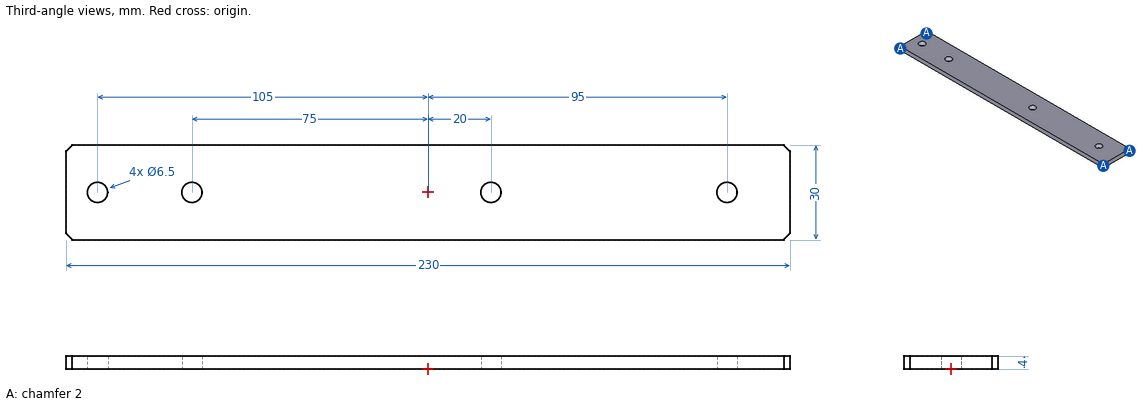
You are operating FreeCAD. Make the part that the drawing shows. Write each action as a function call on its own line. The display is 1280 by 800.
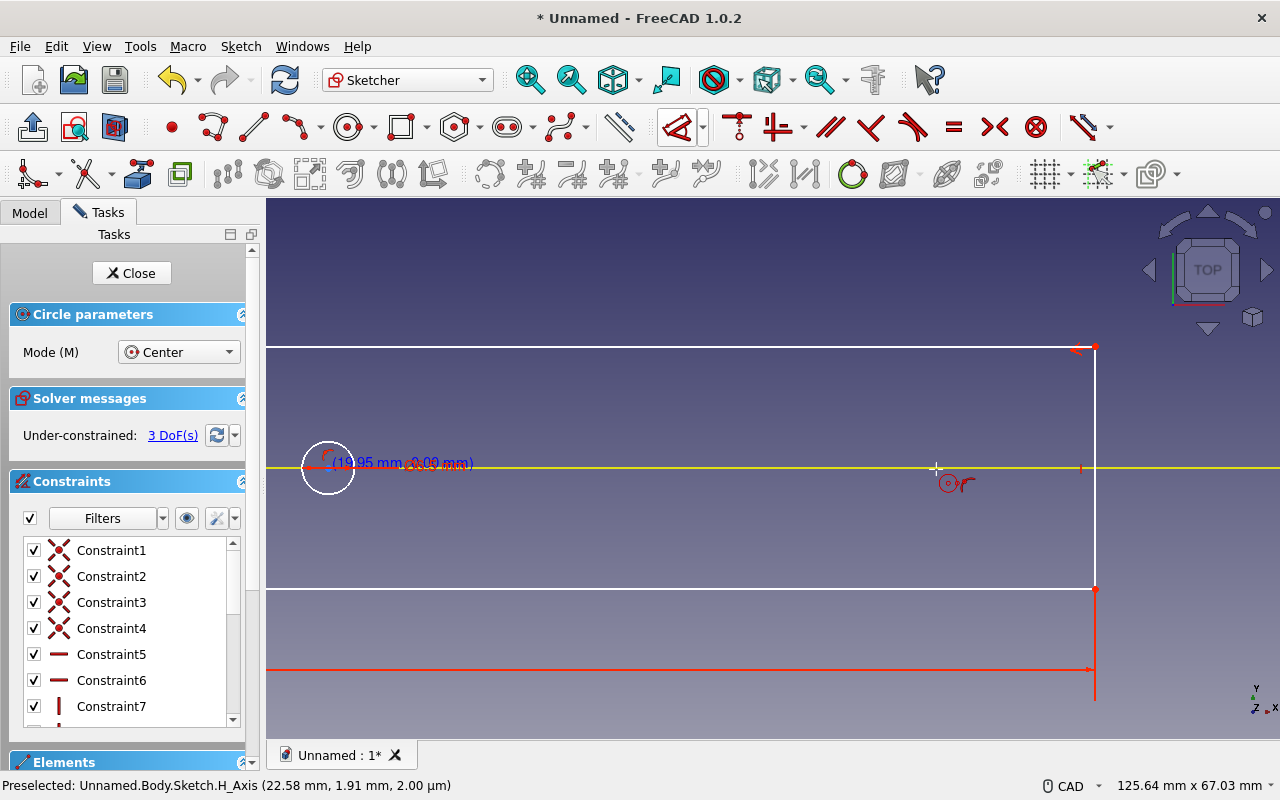
click(934, 468)
move(953, 449)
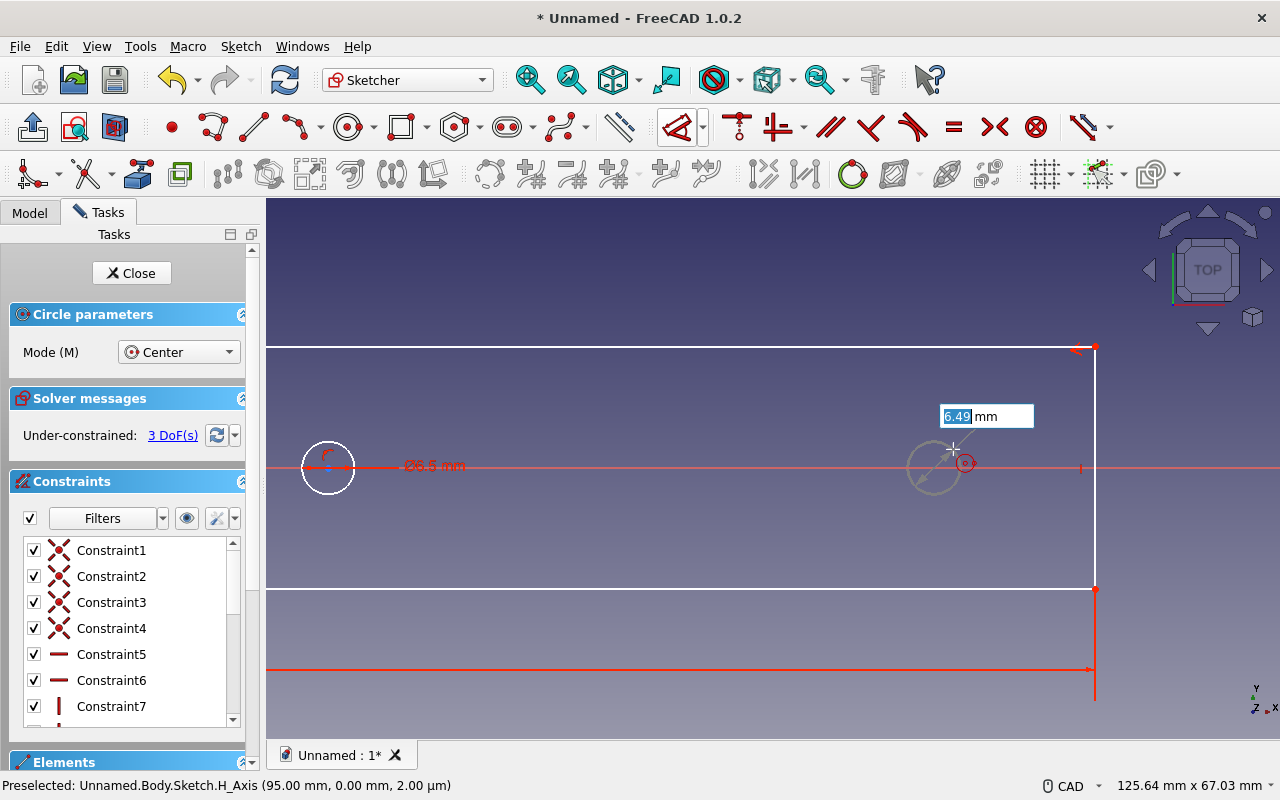
text(6.5)
key(Return)
key(Escape)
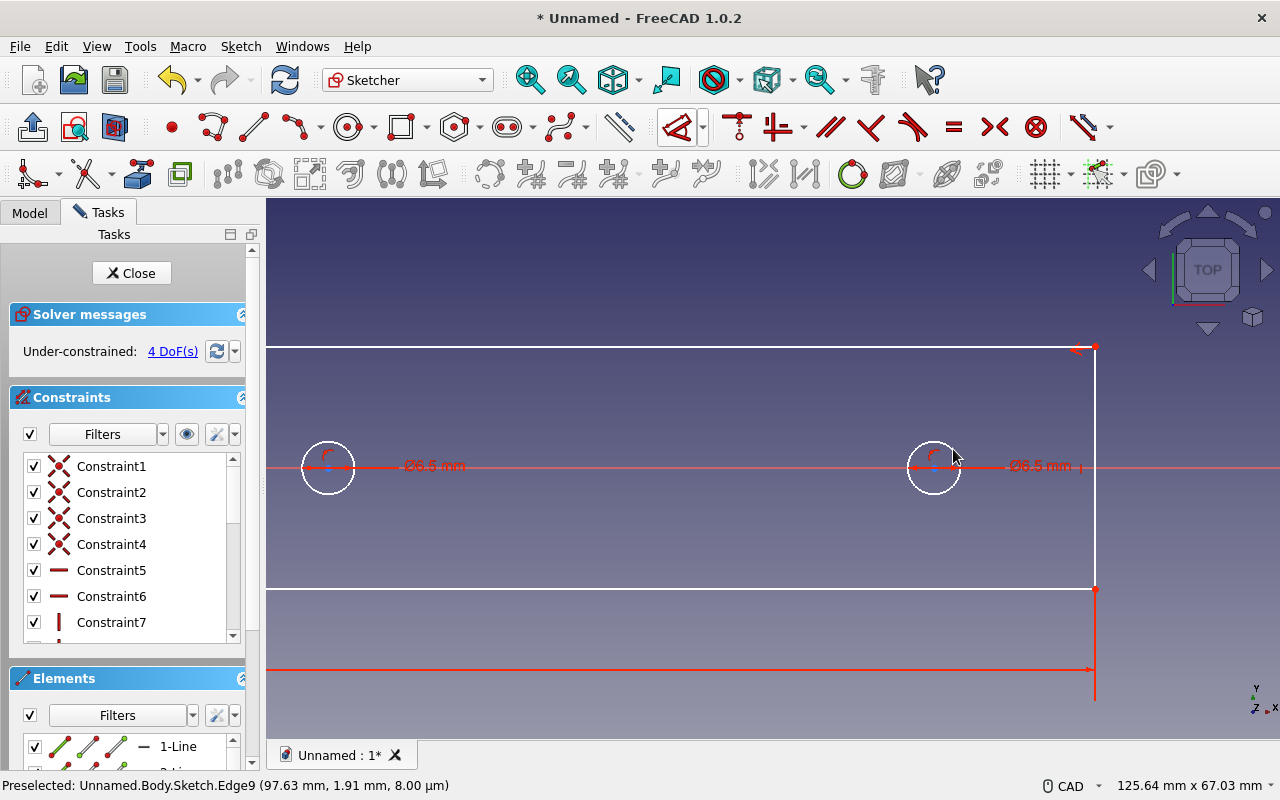
key(d)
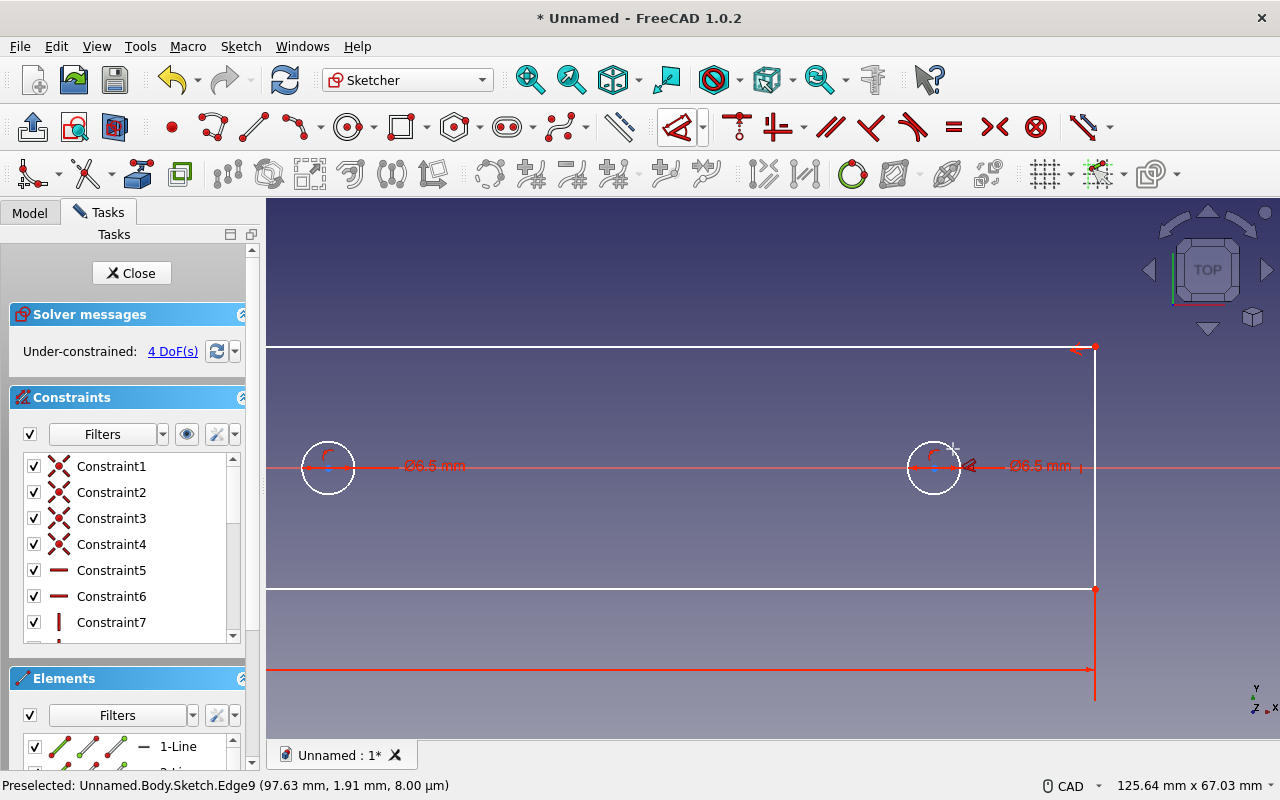
scroll(936, 469, down, 6)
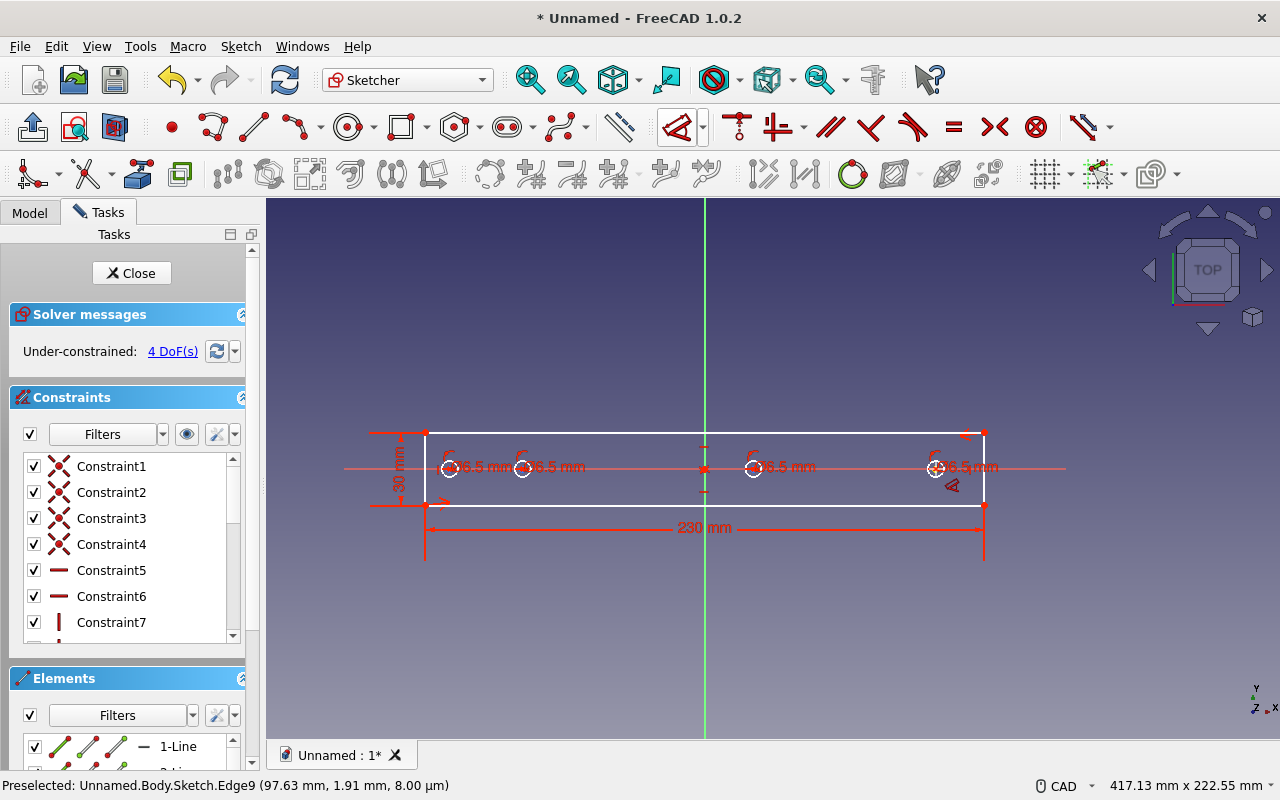
click(523, 469)
click(614, 527)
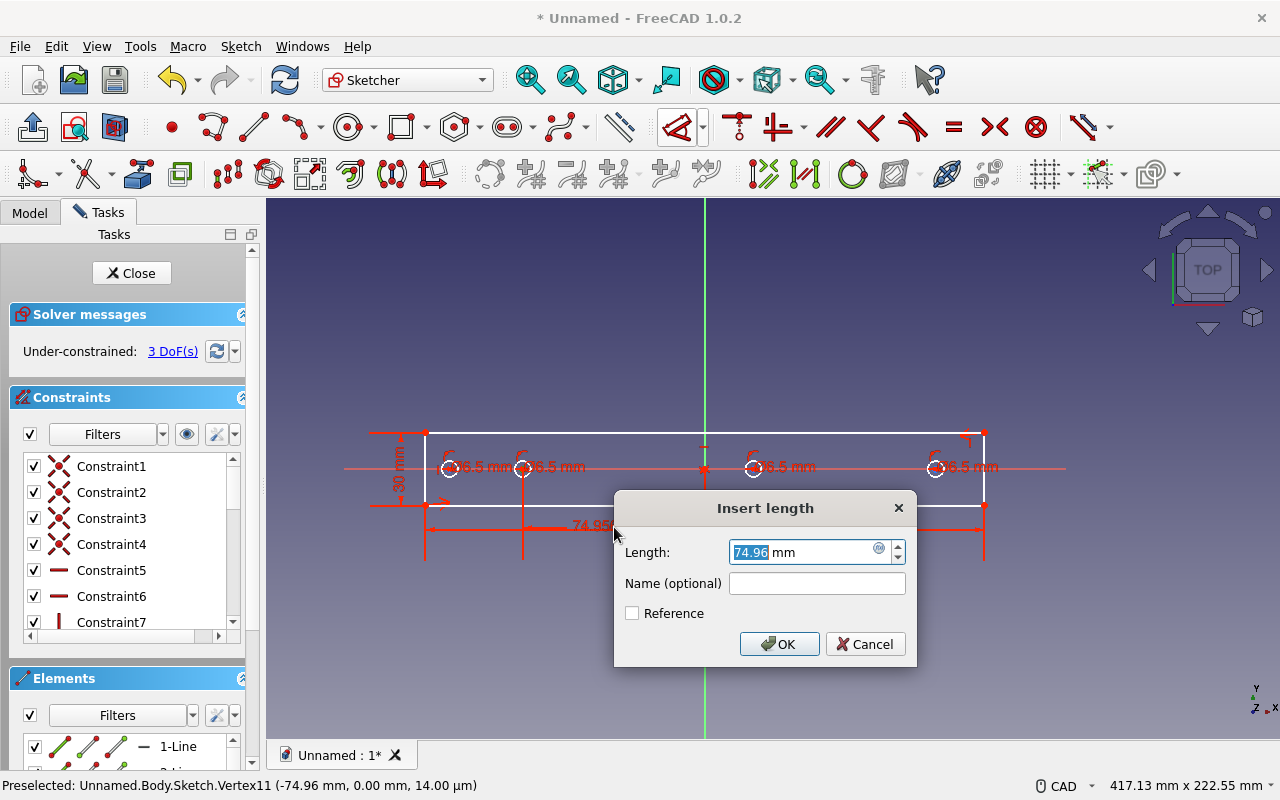
text(75)
key(Return)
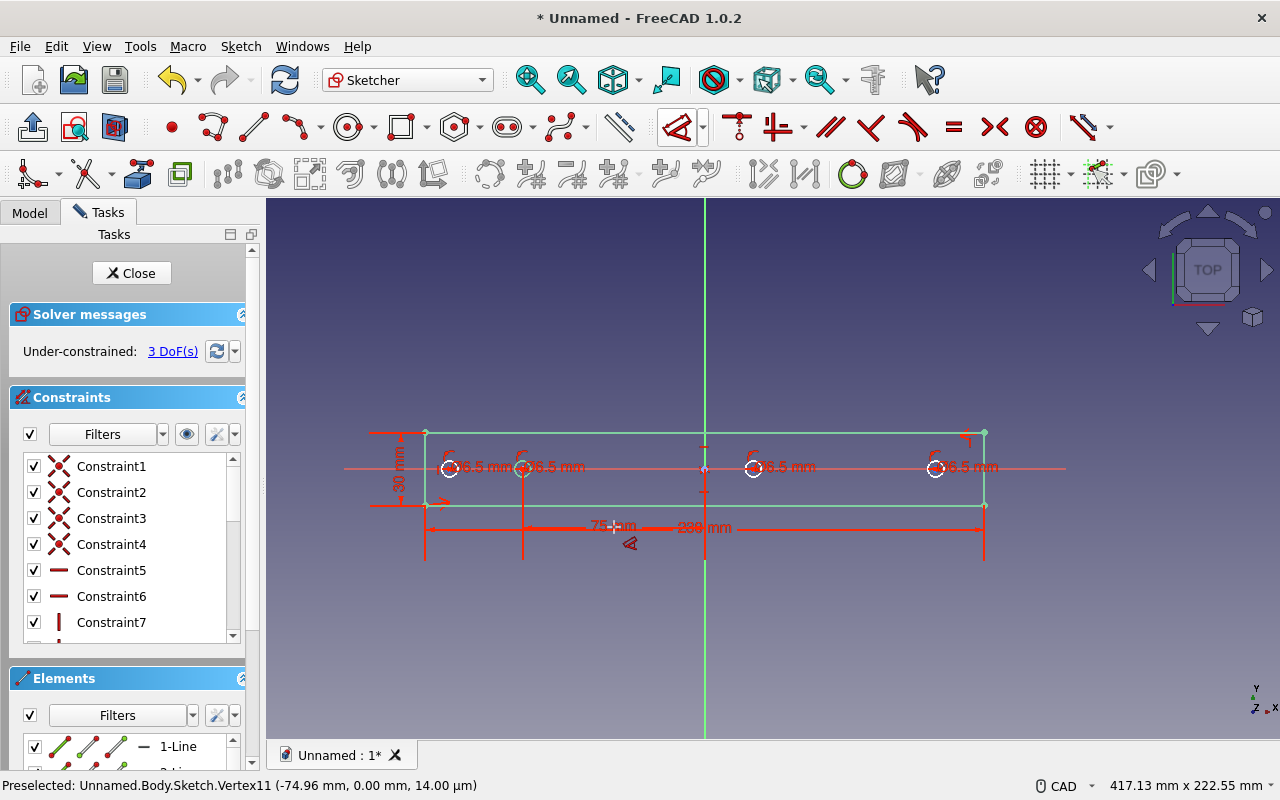
click(753, 469)
click(729, 527)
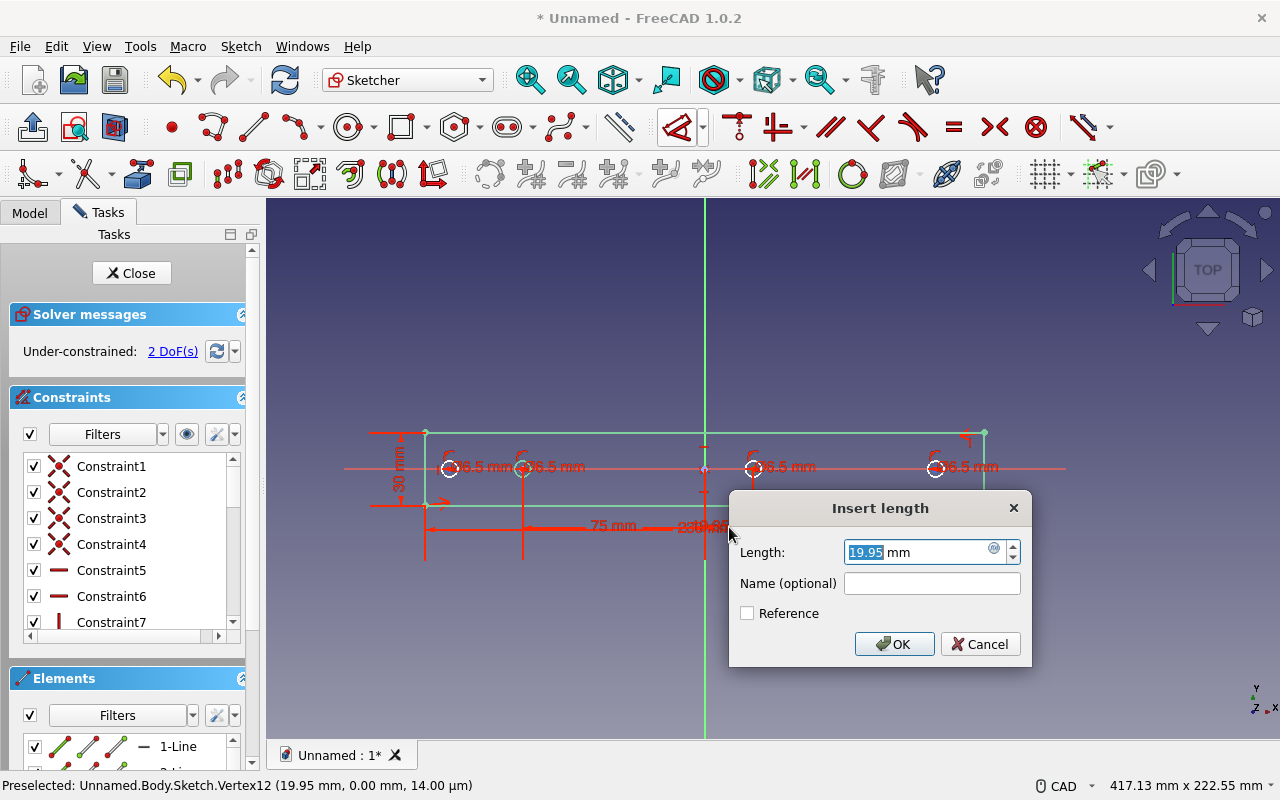
text(20)
key(Return)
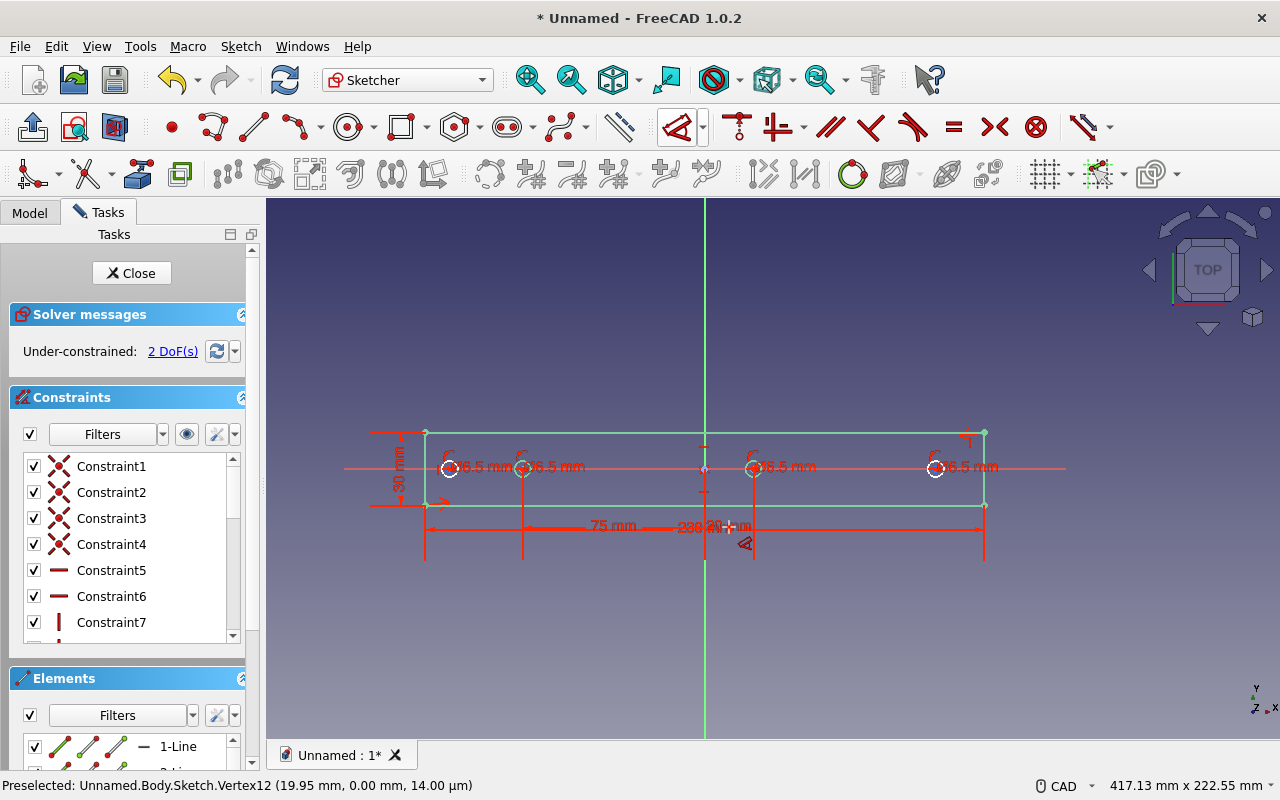
click(936, 469)
click(820, 527)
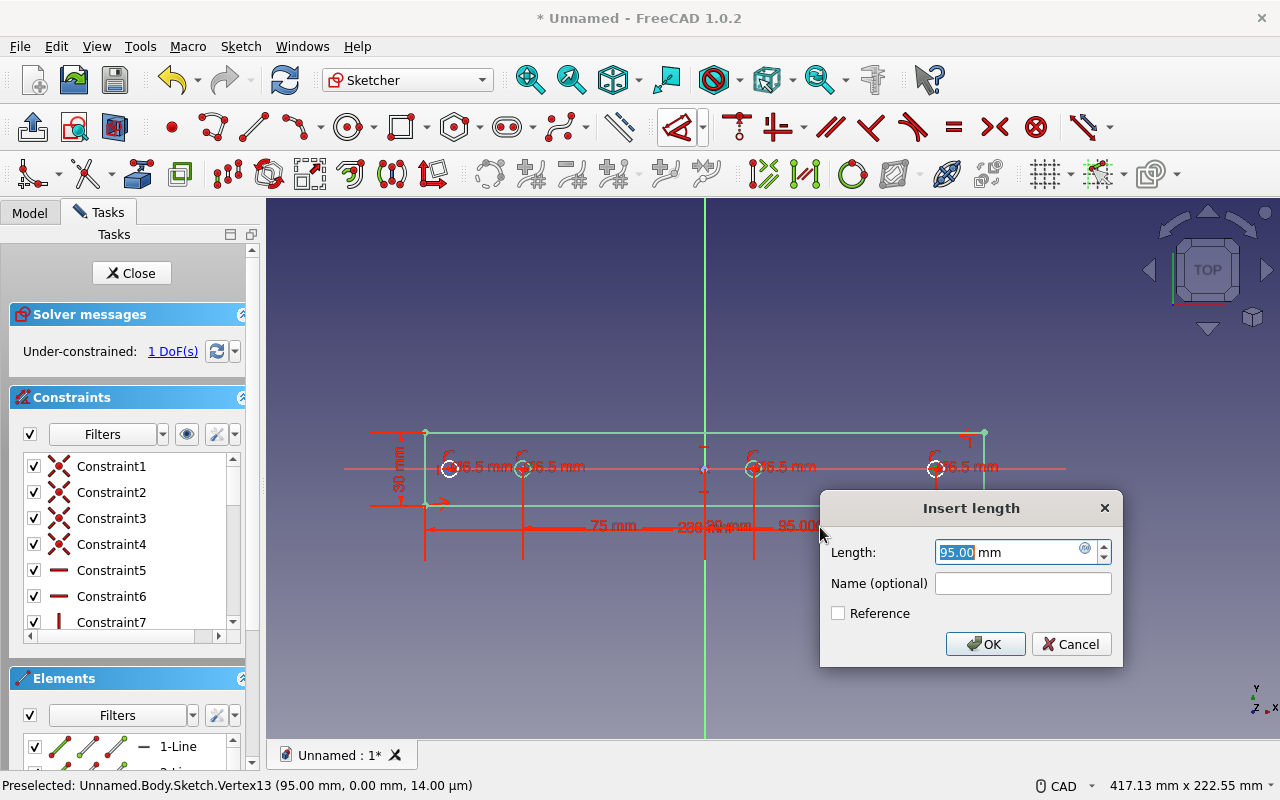
text(95)
key(Return)